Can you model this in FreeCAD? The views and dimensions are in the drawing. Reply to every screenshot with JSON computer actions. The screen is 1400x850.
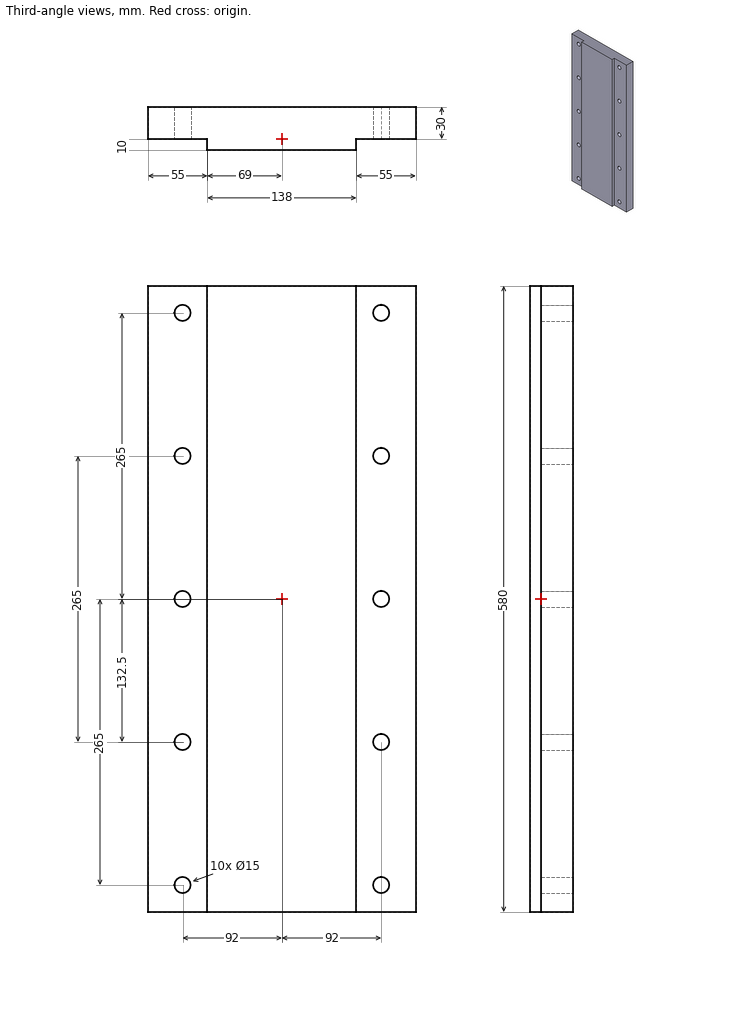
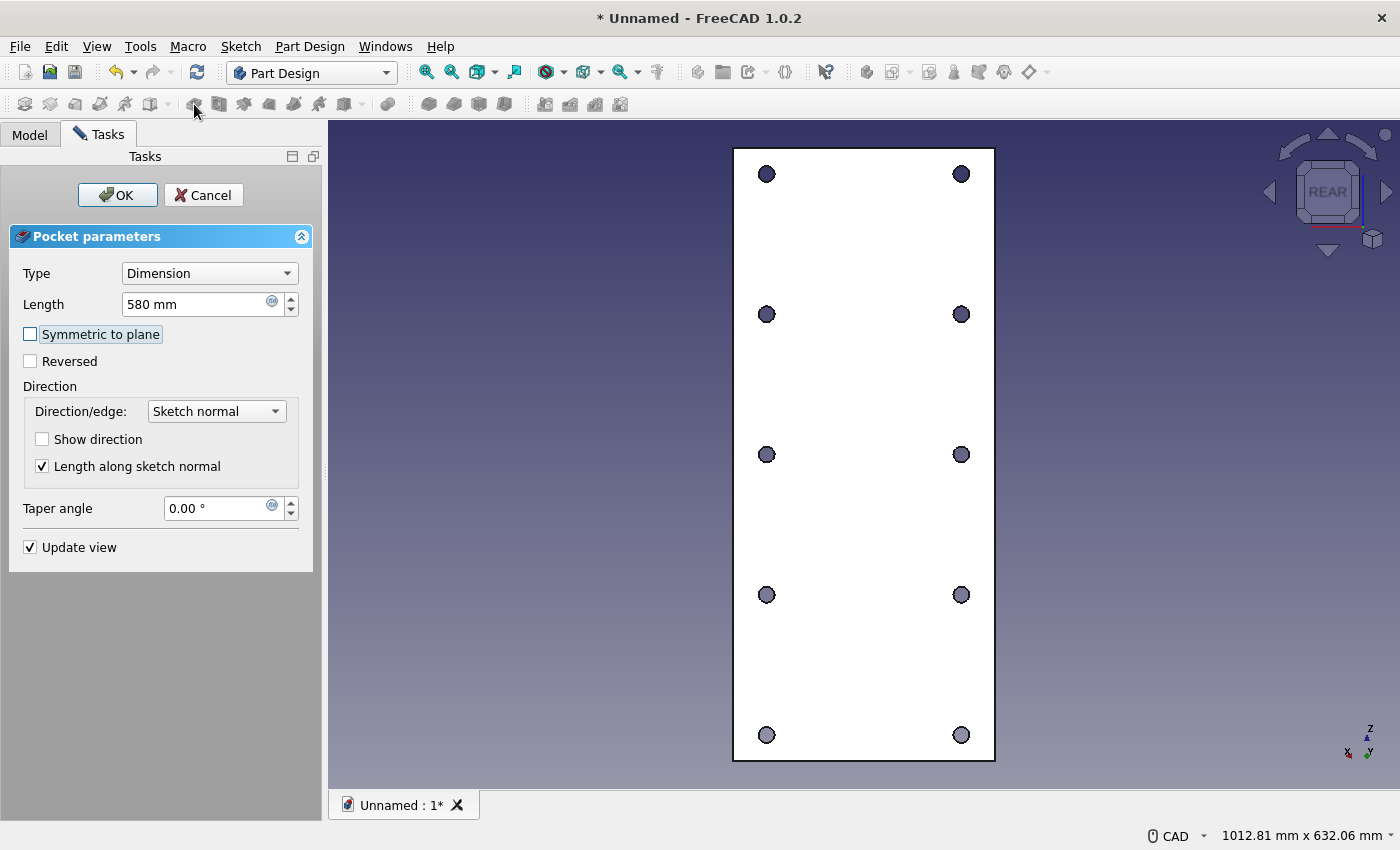
{"action": "left_click", "coordinate": [31, 334]}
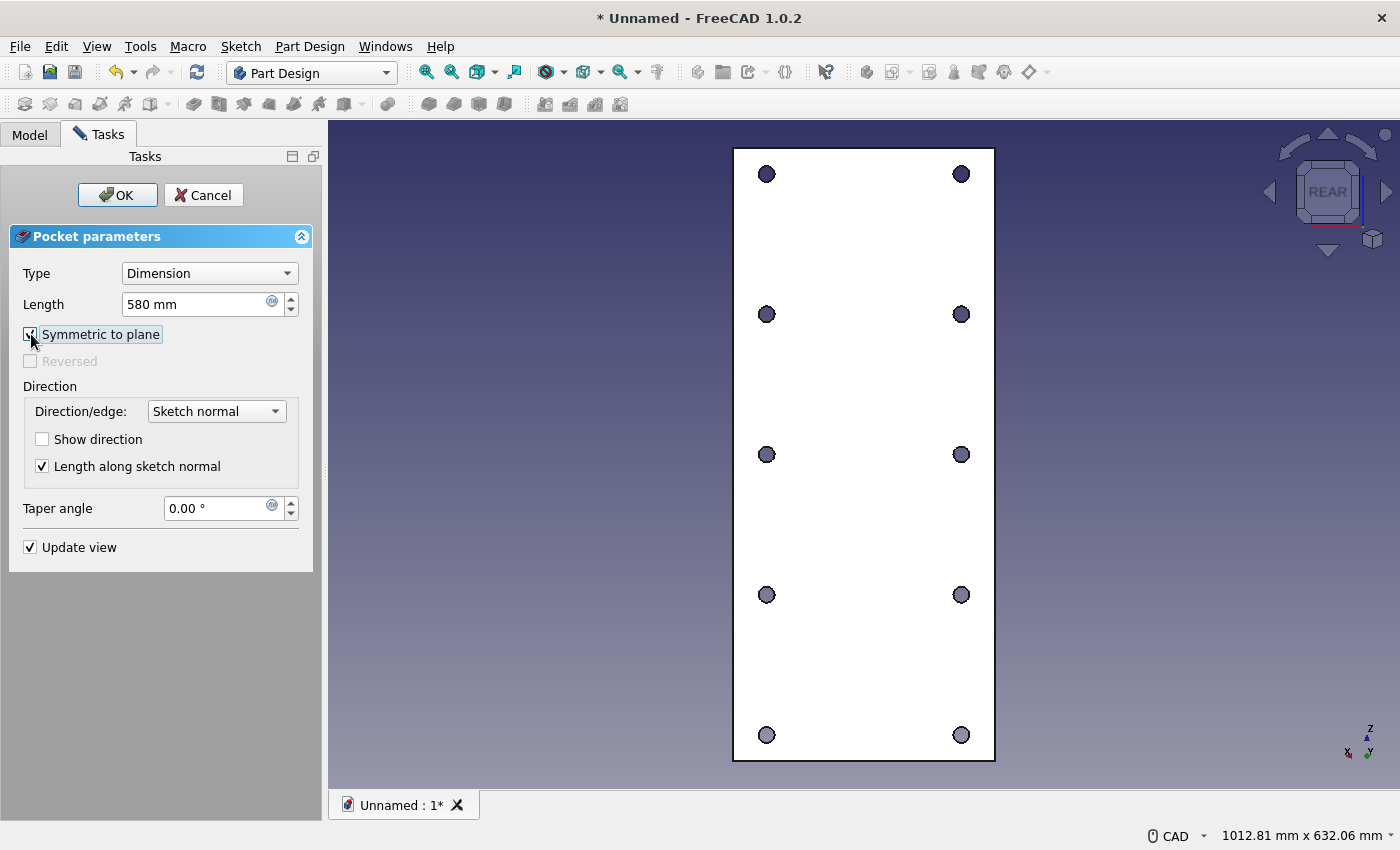
{"action": "left_click", "coordinate": [118, 195]}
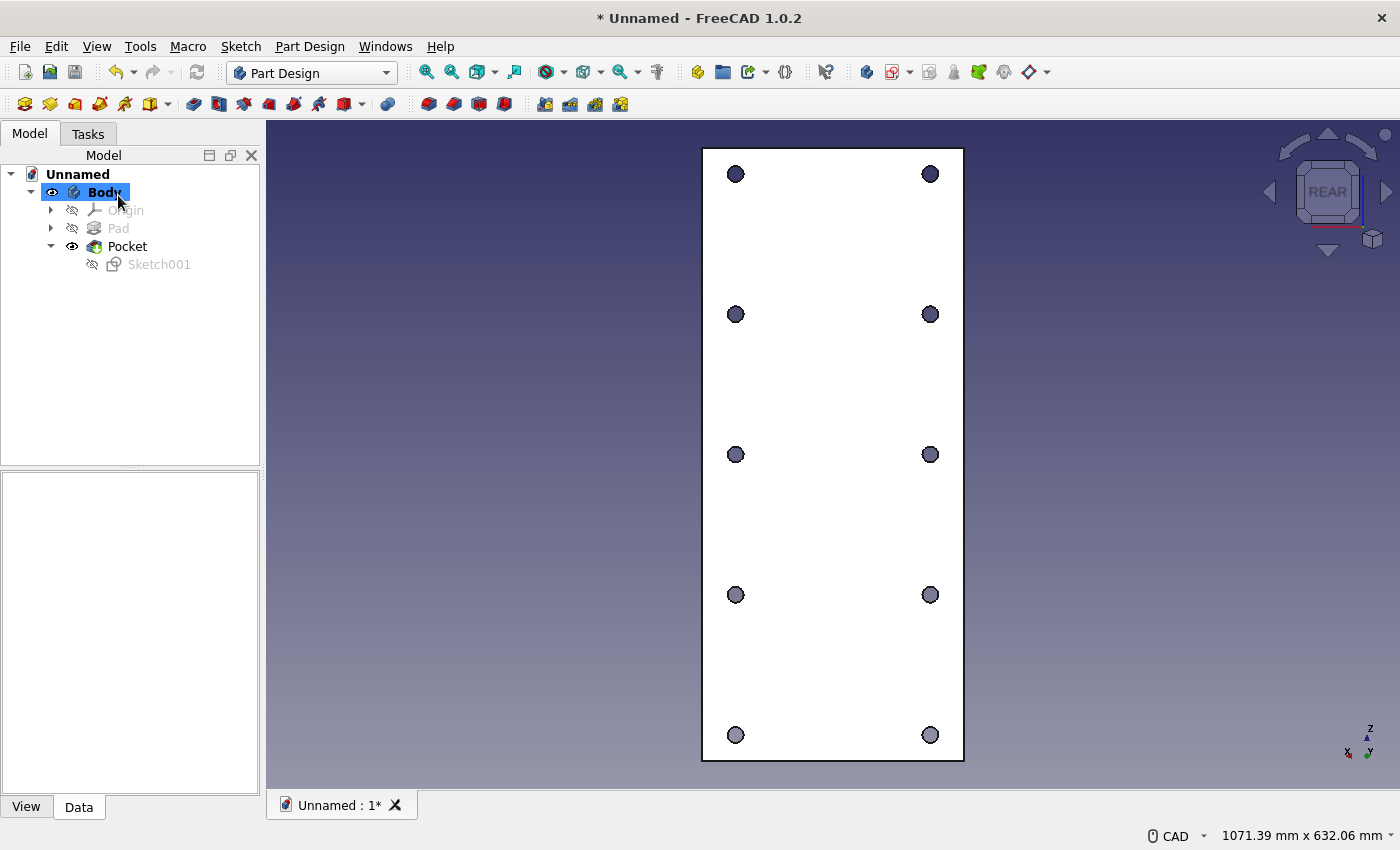
{"action": "key", "text": "0"}